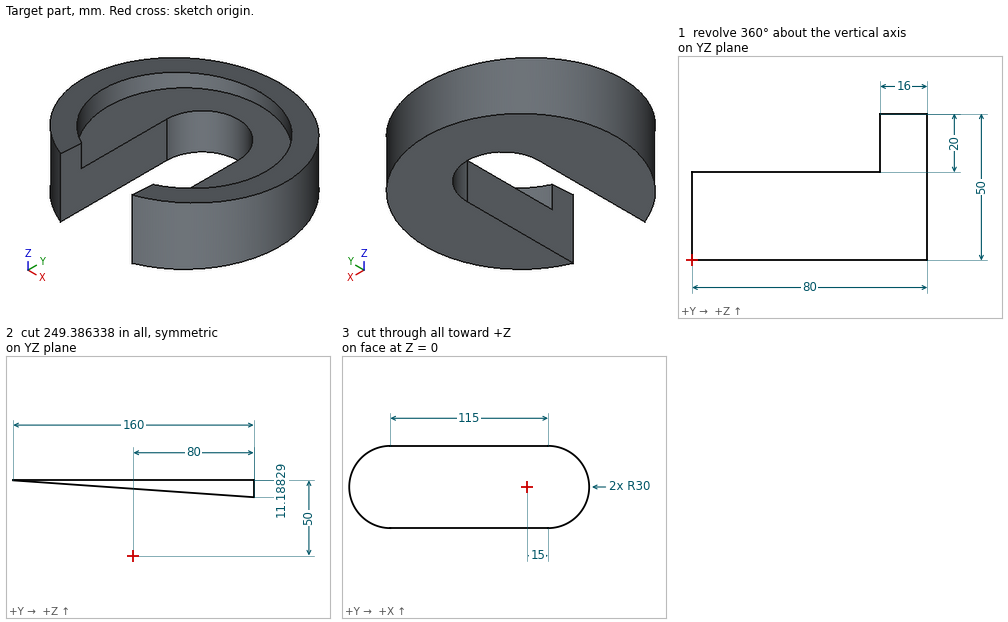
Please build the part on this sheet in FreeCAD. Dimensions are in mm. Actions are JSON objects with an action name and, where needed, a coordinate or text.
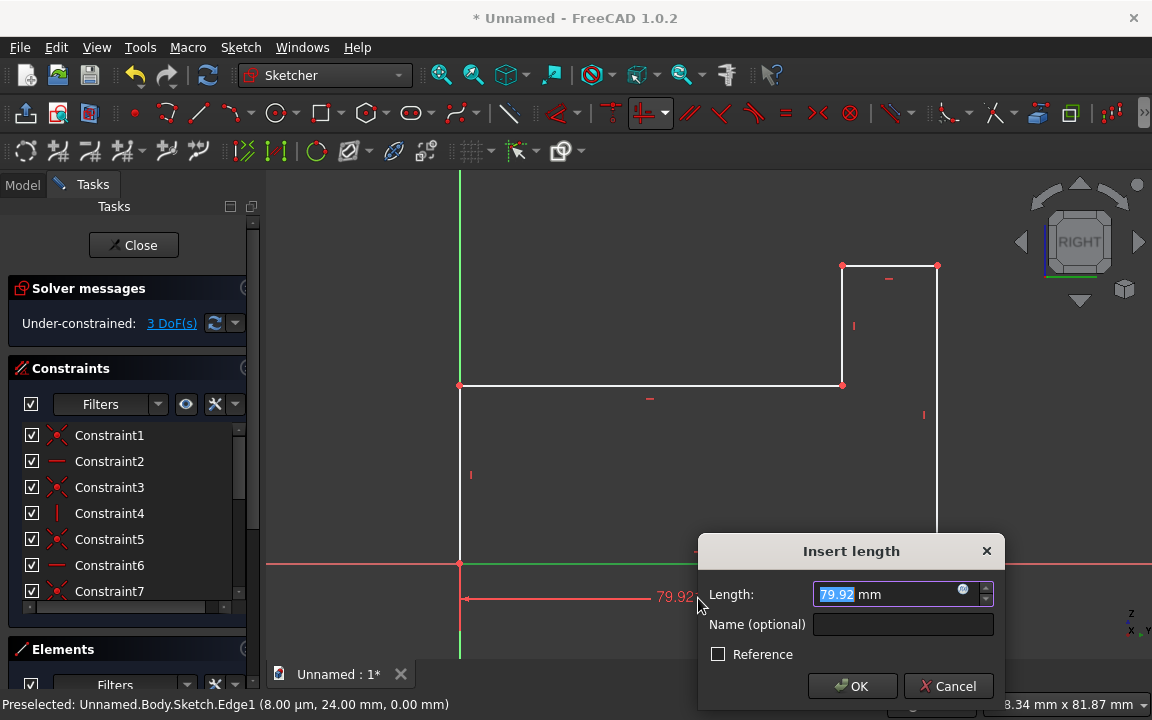
{"action": "type", "text": "80"}
{"action": "key", "text": "Return"}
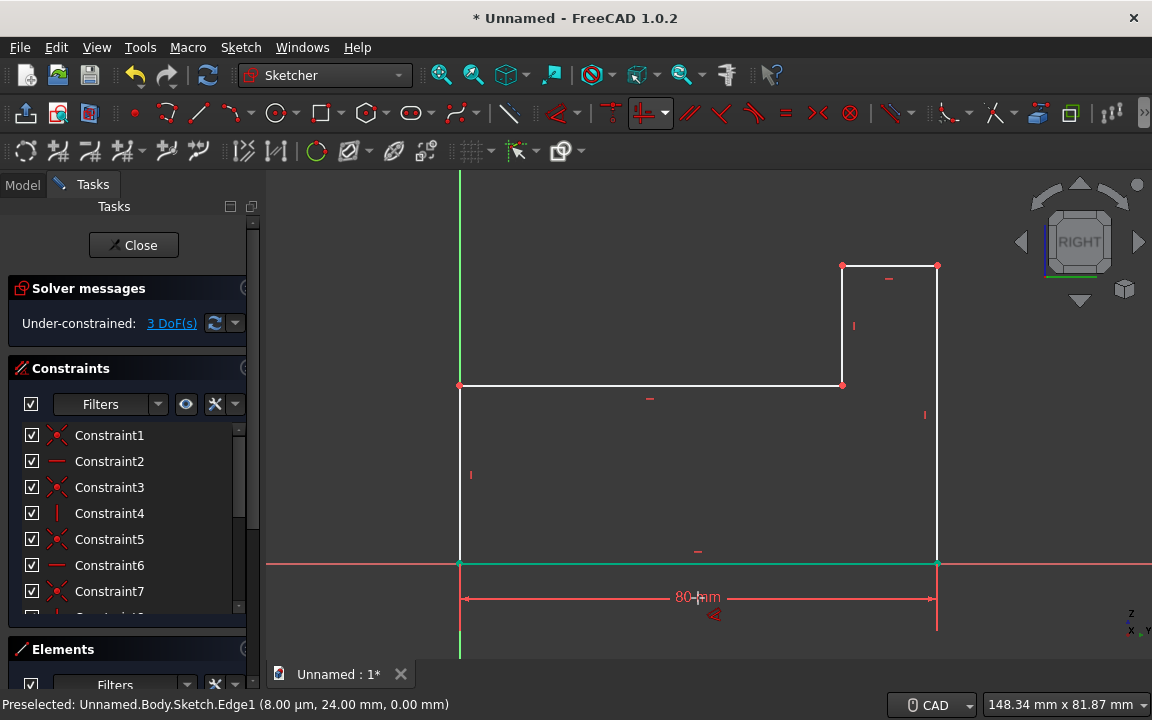
{"action": "left_click", "coordinate": [937, 475]}
{"action": "left_click", "coordinate": [971, 415]}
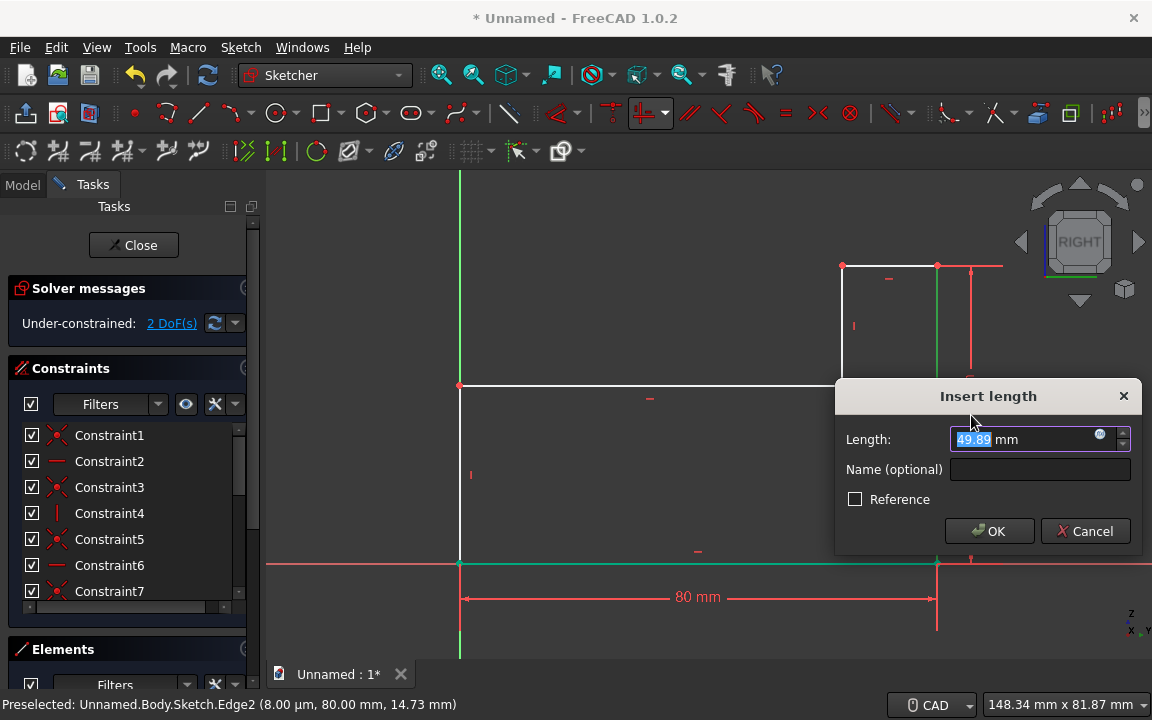
{"action": "type", "text": "50"}
{"action": "key", "text": "Return"}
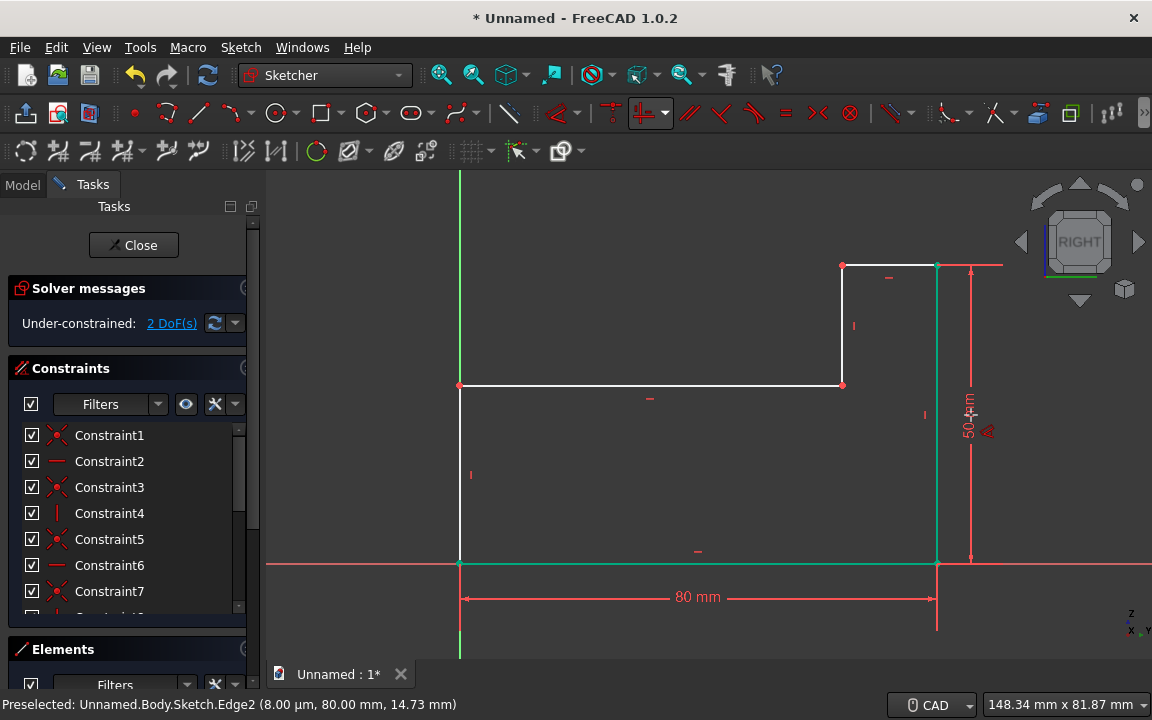
{"action": "left_click", "coordinate": [909, 265]}
{"action": "left_click", "coordinate": [890, 231]}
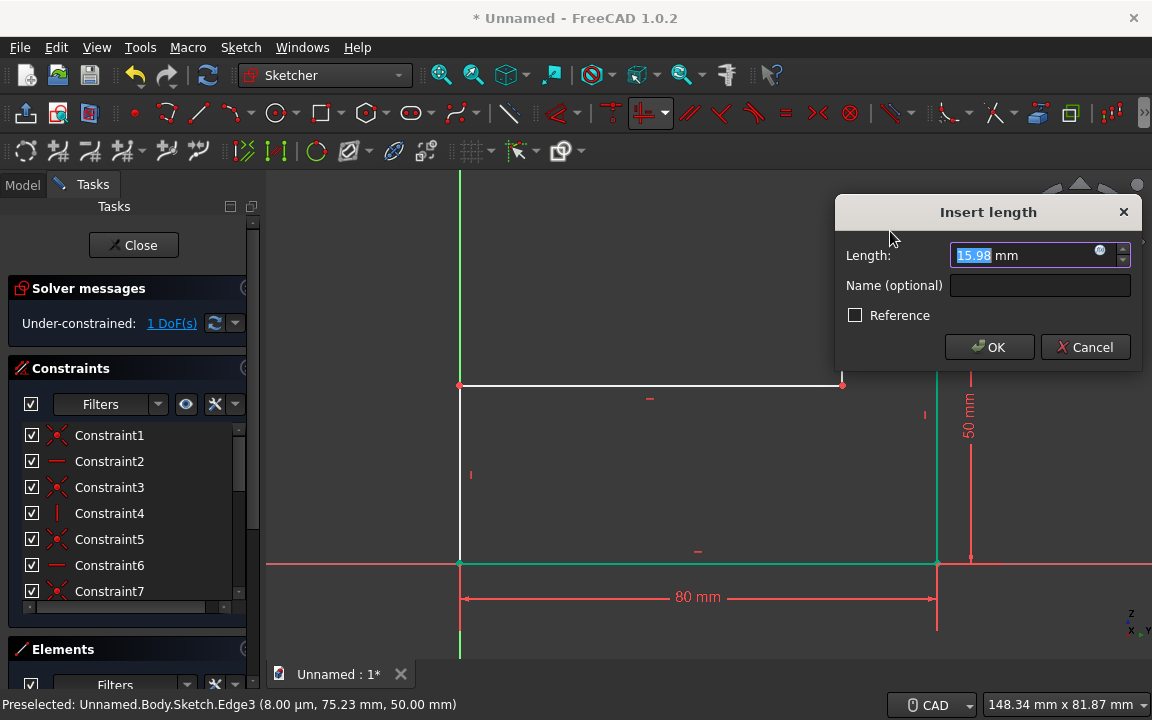
{"action": "type", "text": "16"}
{"action": "key", "text": "Return"}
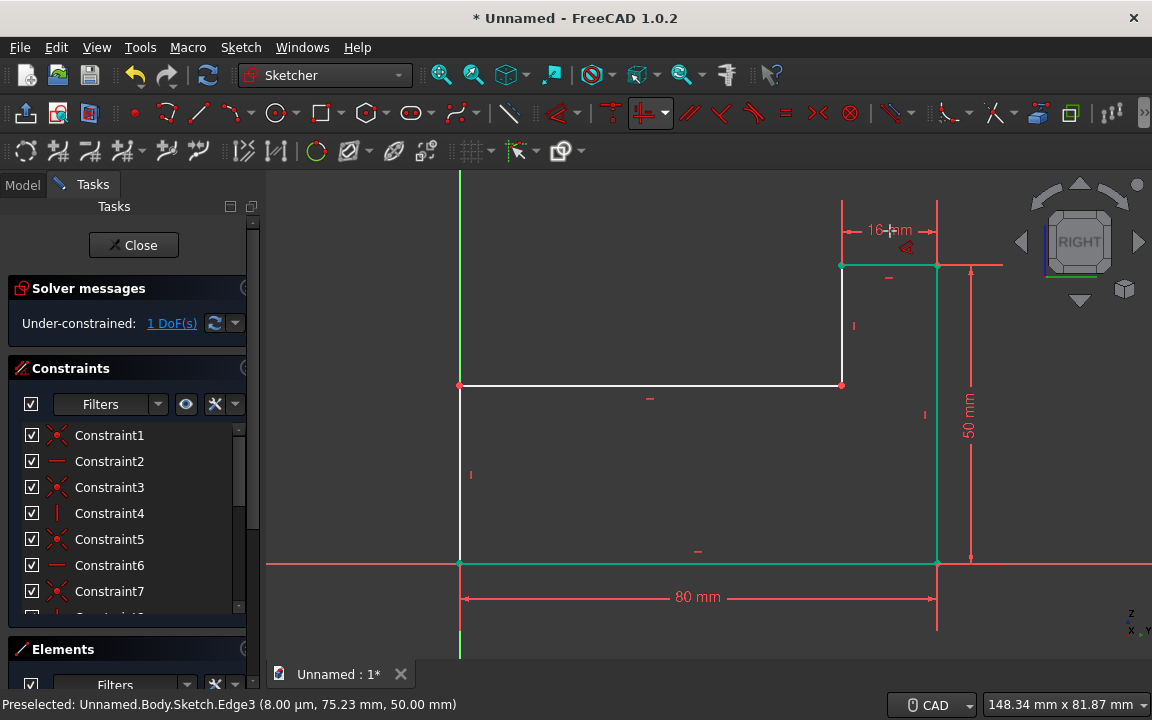
{"action": "left_click", "coordinate": [842, 302]}
{"action": "left_click", "coordinate": [876, 326]}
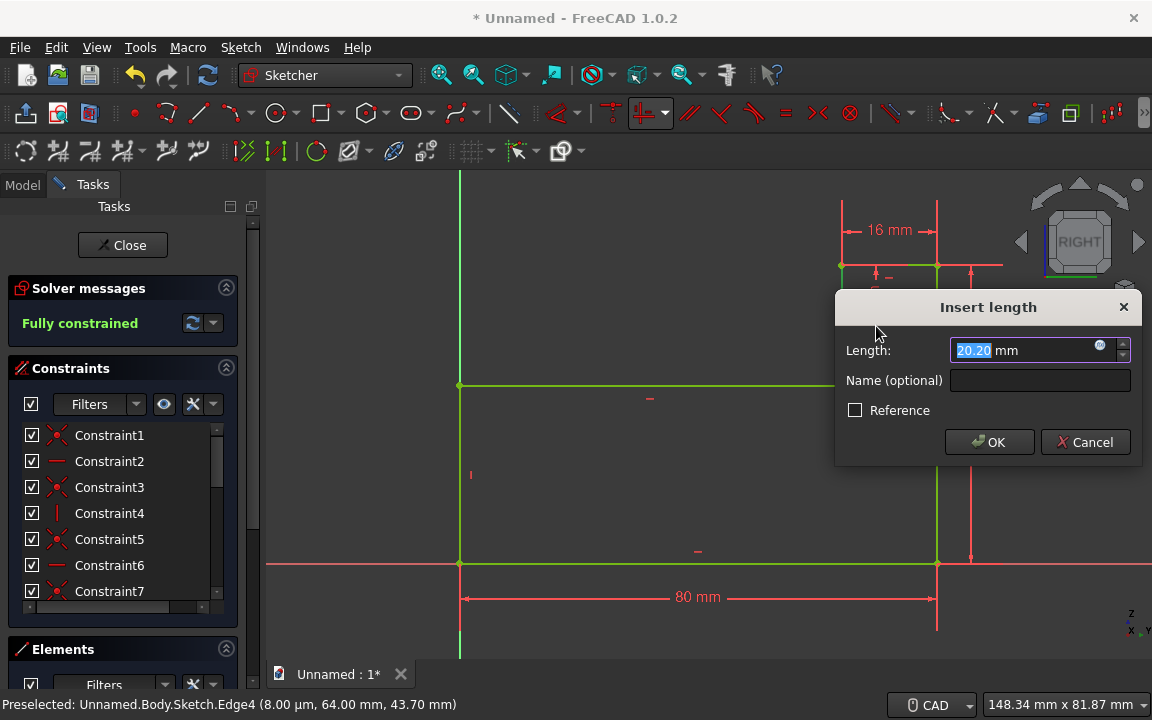
{"action": "type", "text": "20"}
{"action": "key", "text": "Return"}
{"action": "key", "text": "Escape"}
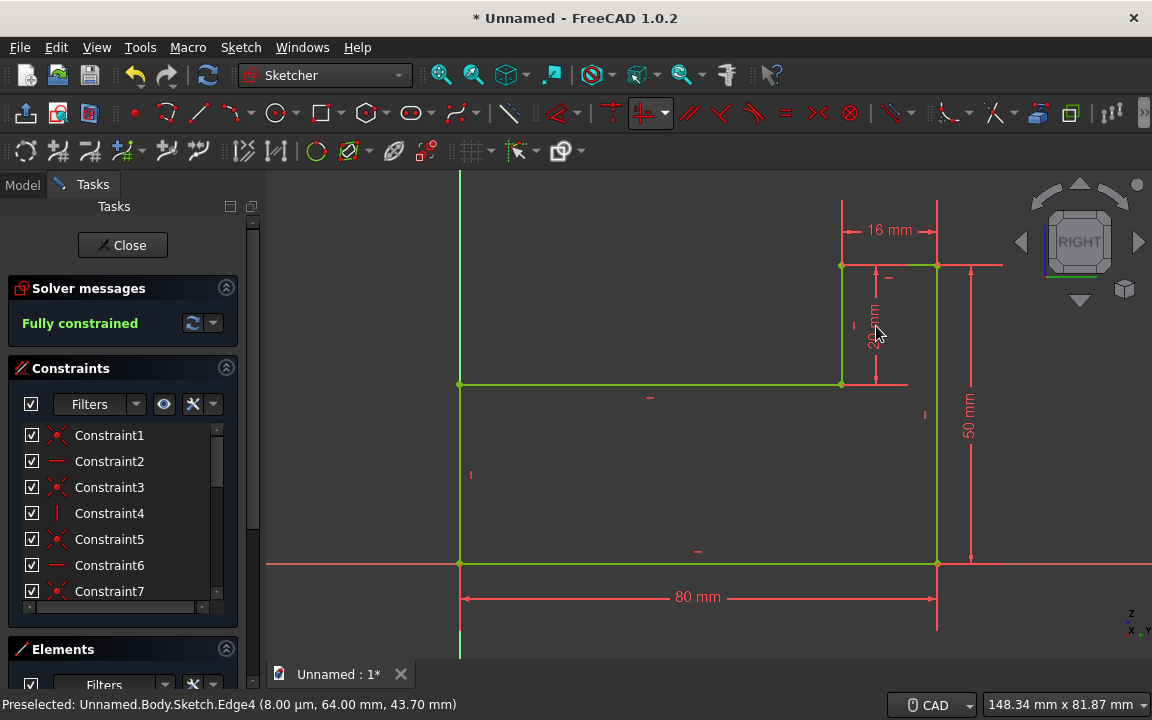
{"action": "left_click", "coordinate": [123, 245]}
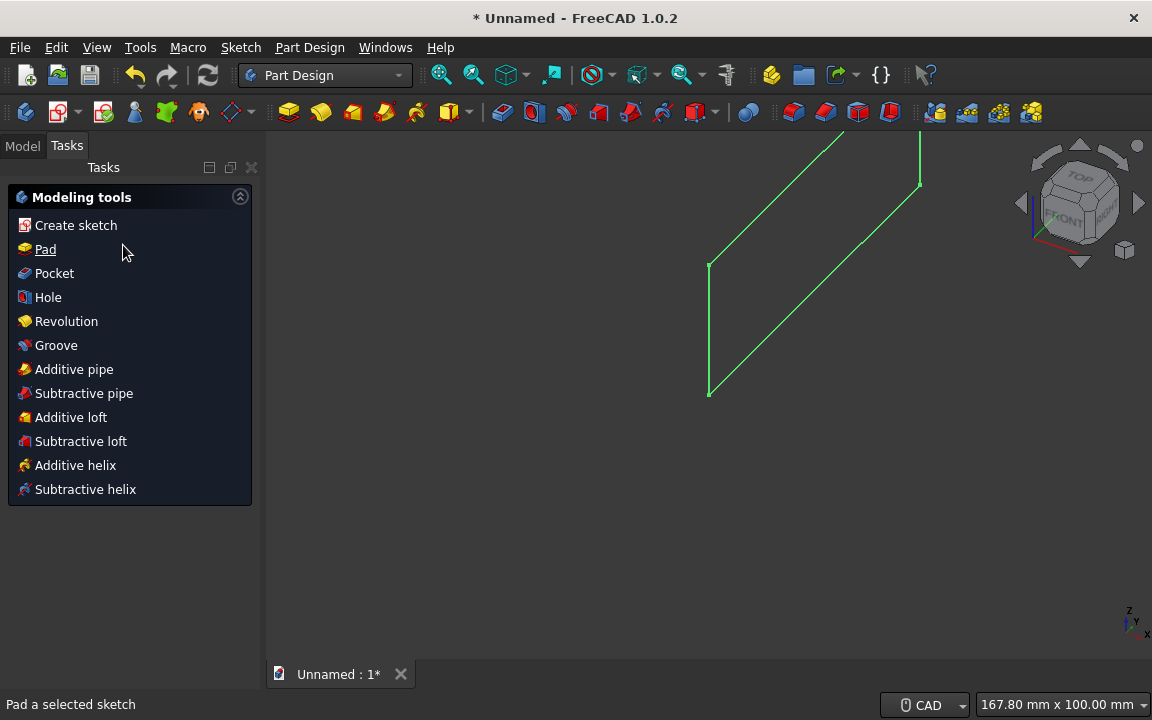
{"action": "left_click", "coordinate": [322, 112]}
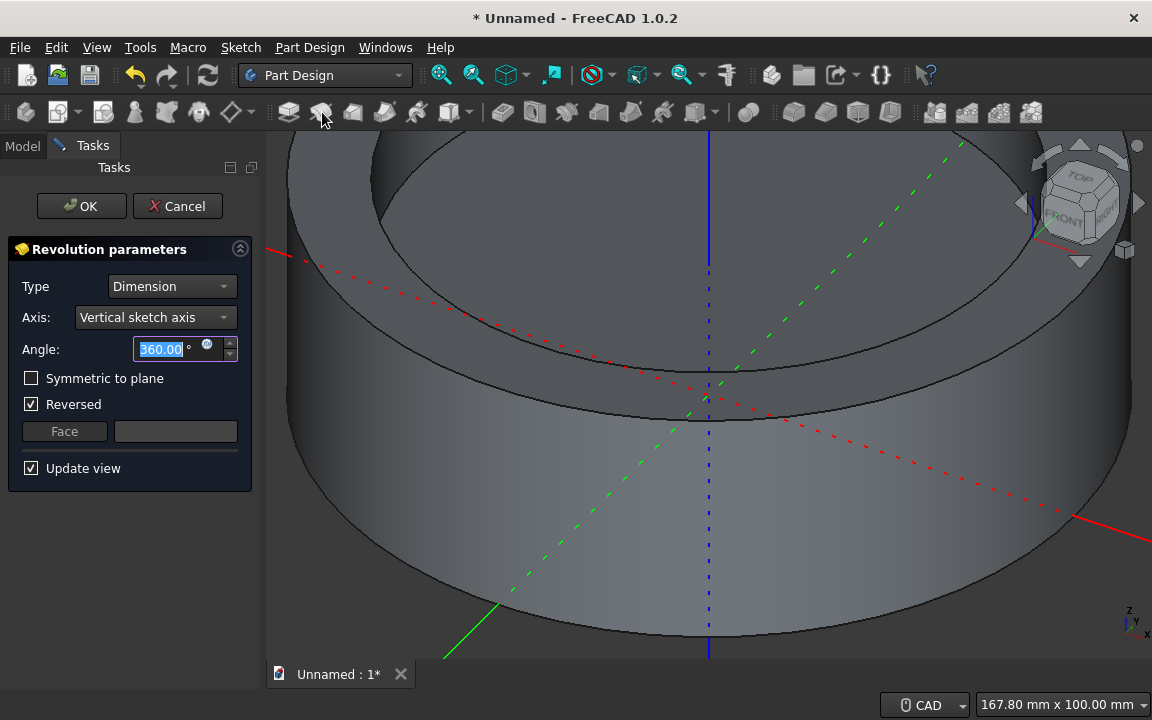
{"action": "left_click", "coordinate": [82, 206]}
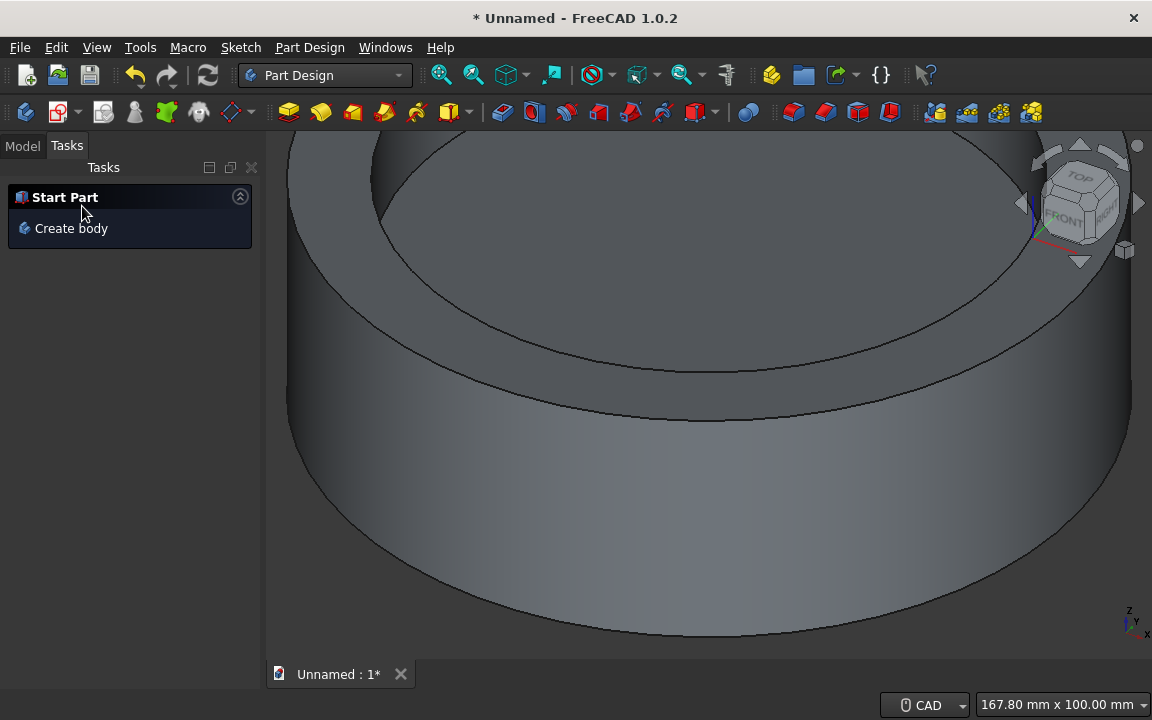
{"action": "left_click", "coordinate": [442, 76]}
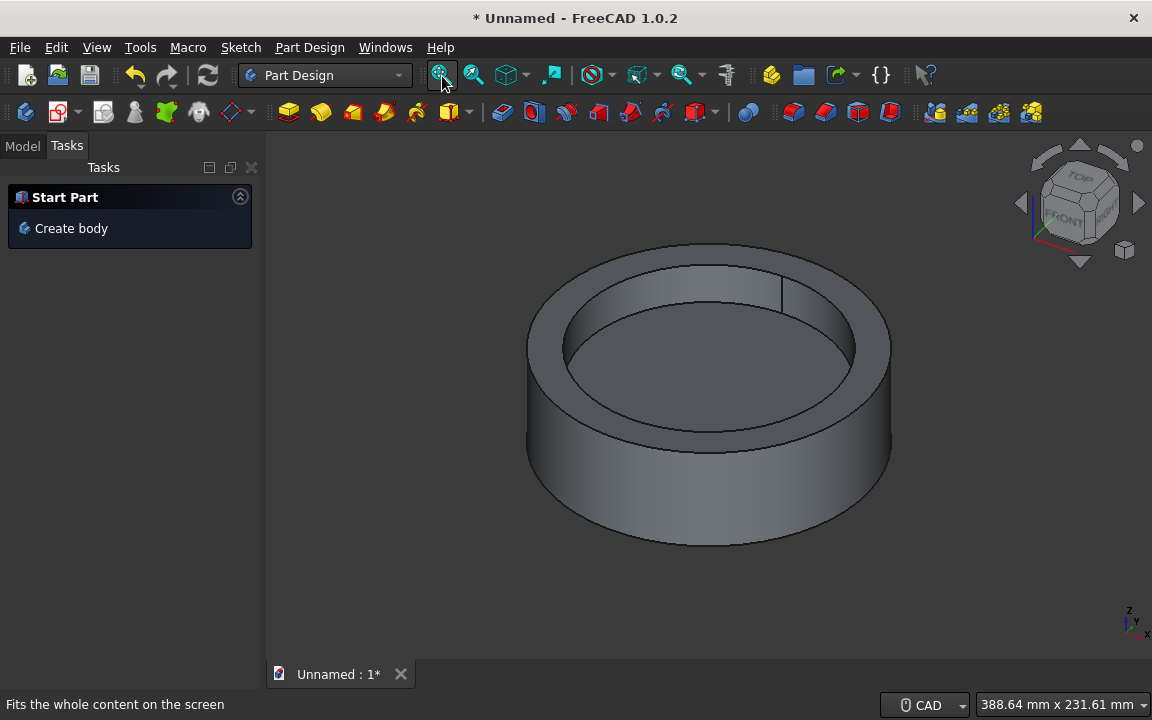
{"action": "left_click", "coordinate": [58, 112]}